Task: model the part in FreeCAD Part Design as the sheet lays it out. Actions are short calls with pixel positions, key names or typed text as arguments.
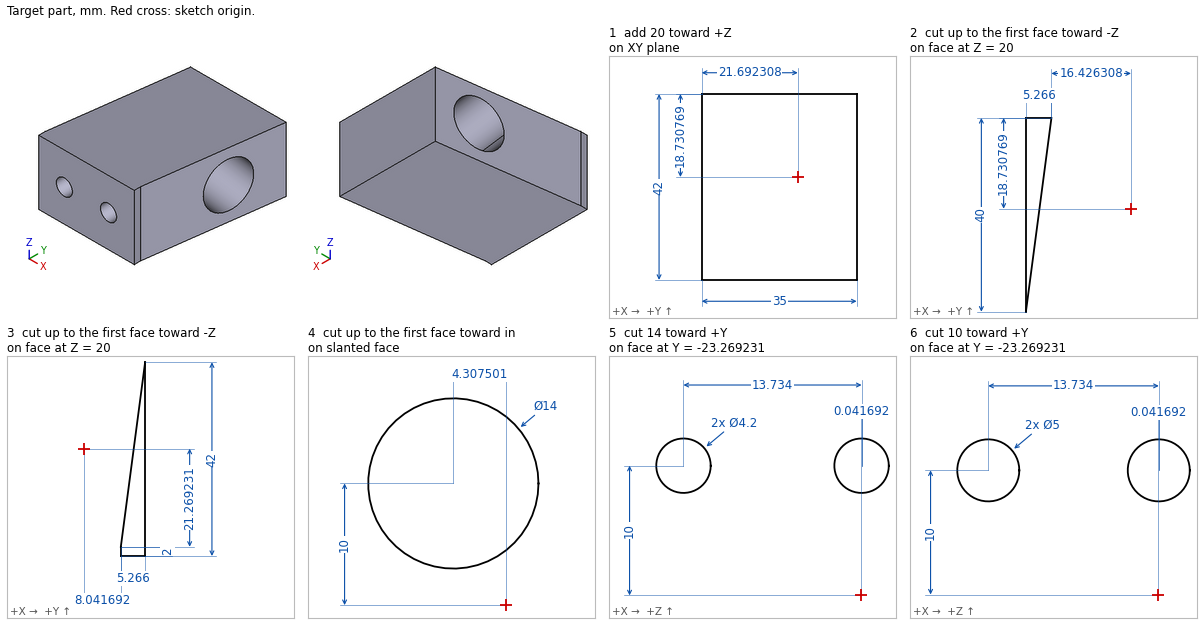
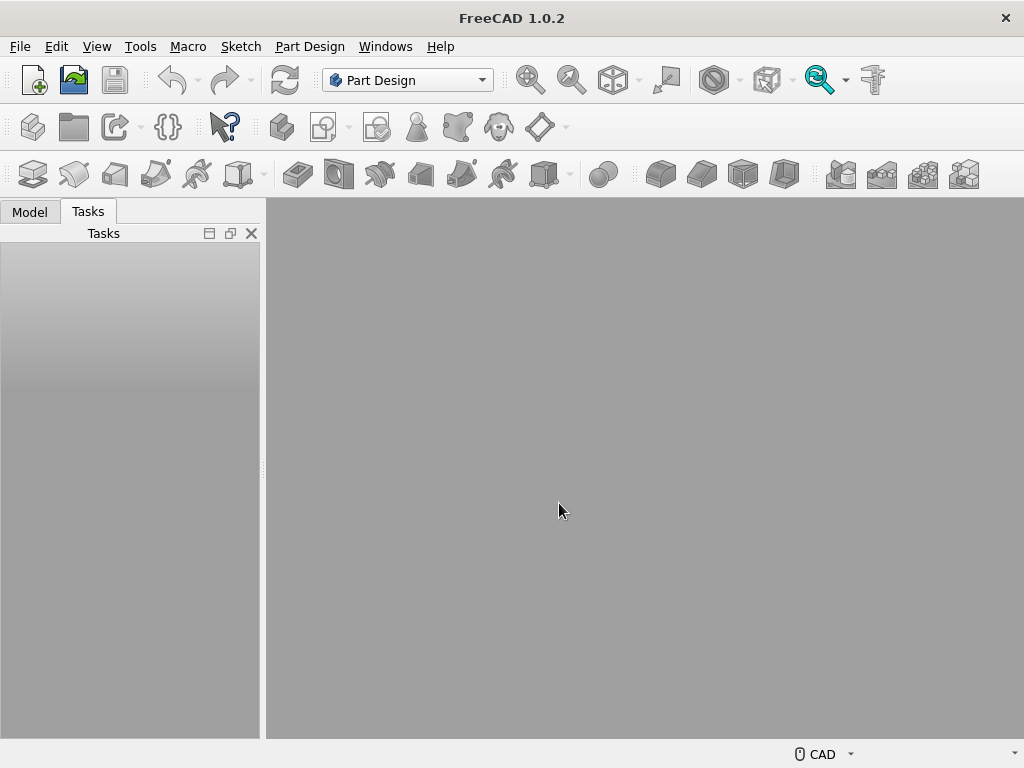
click(33, 80)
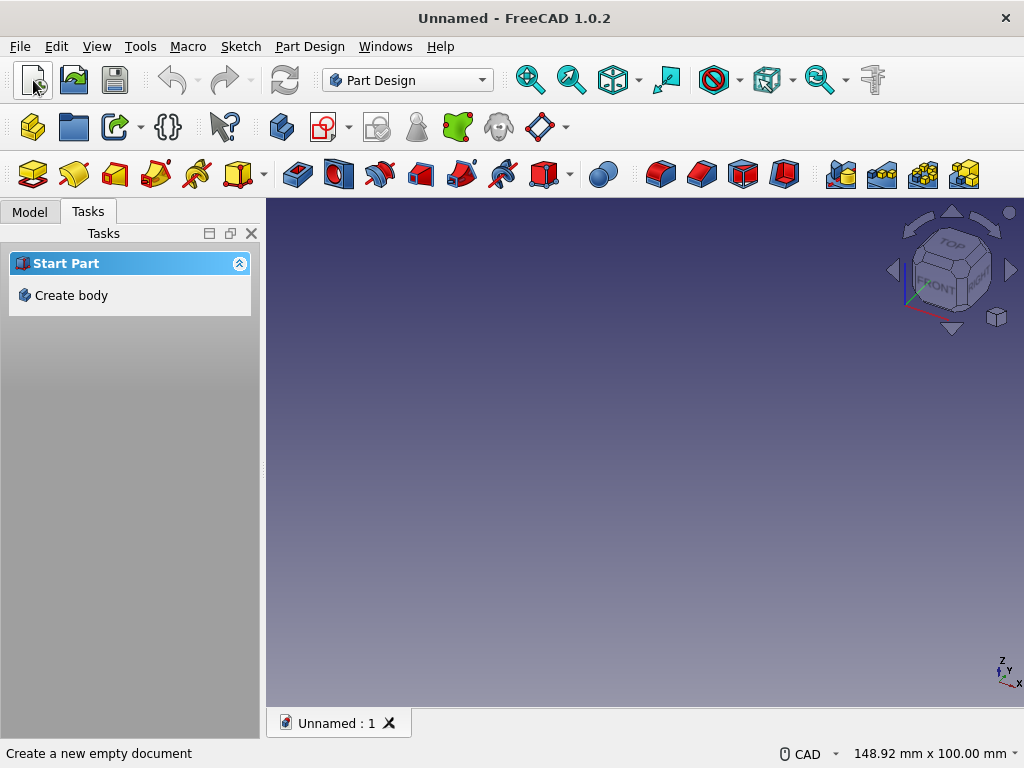
click(322, 128)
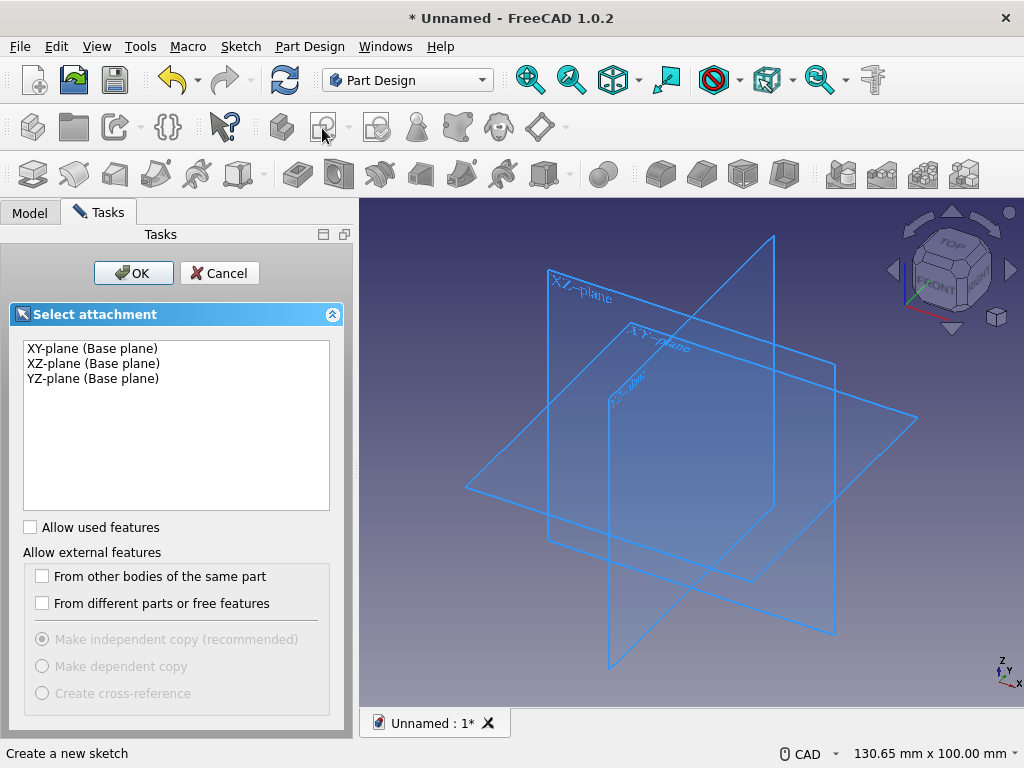
click(84, 348)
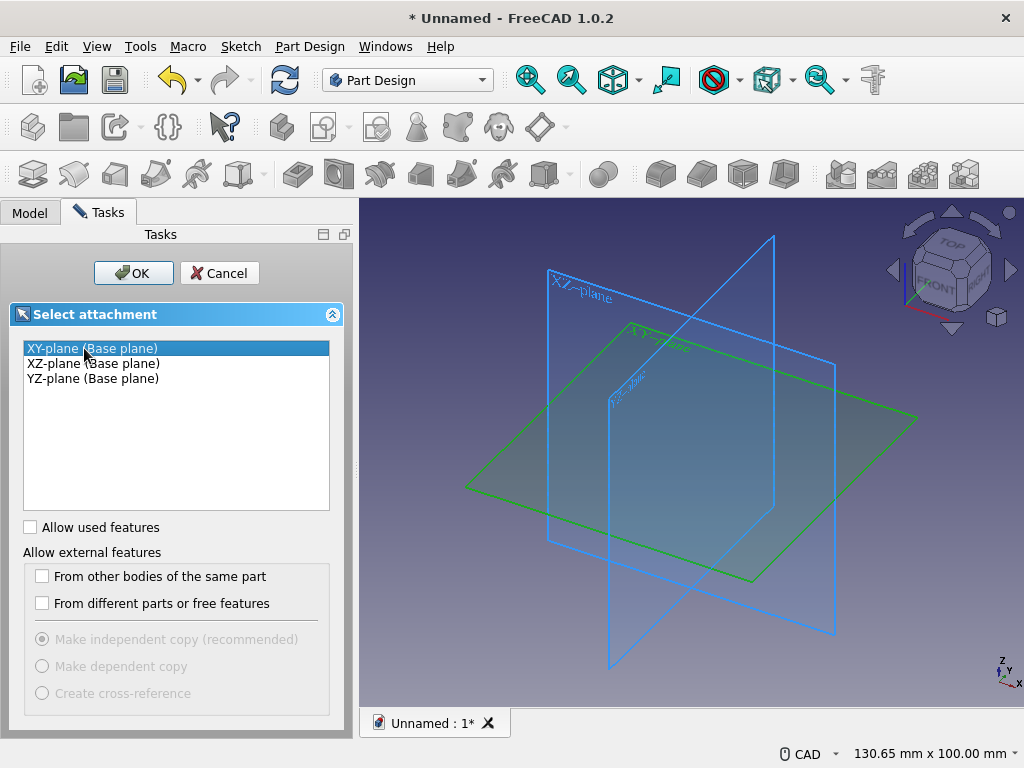
click(134, 273)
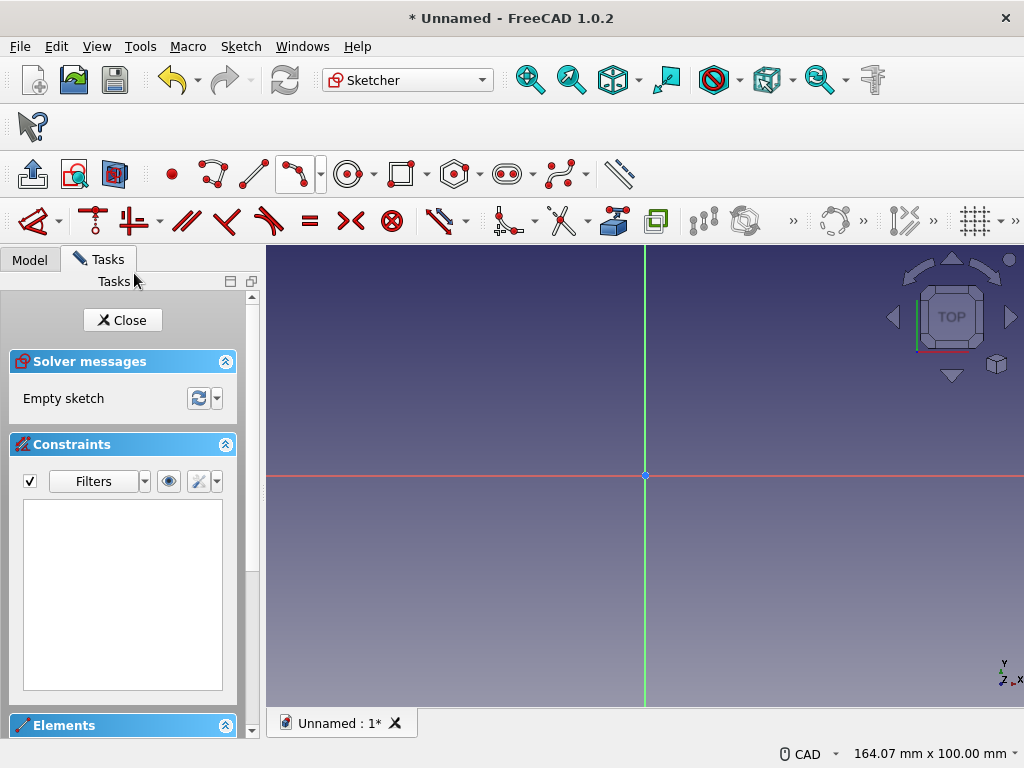
scroll(726, 508, up, 2)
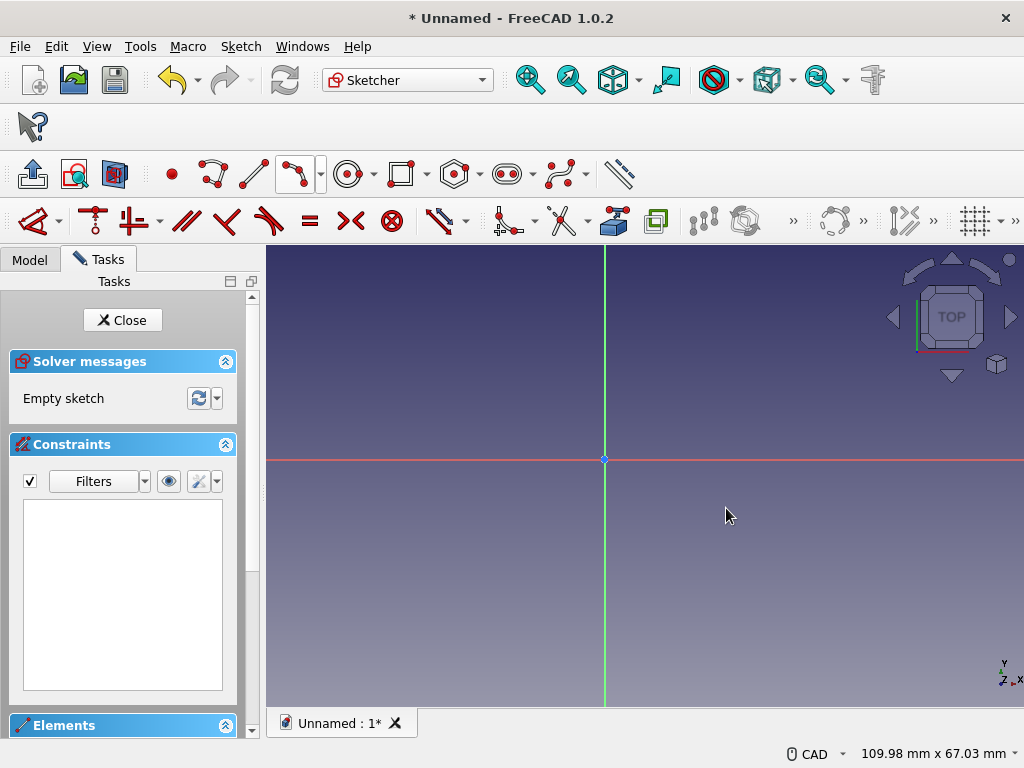
click(400, 174)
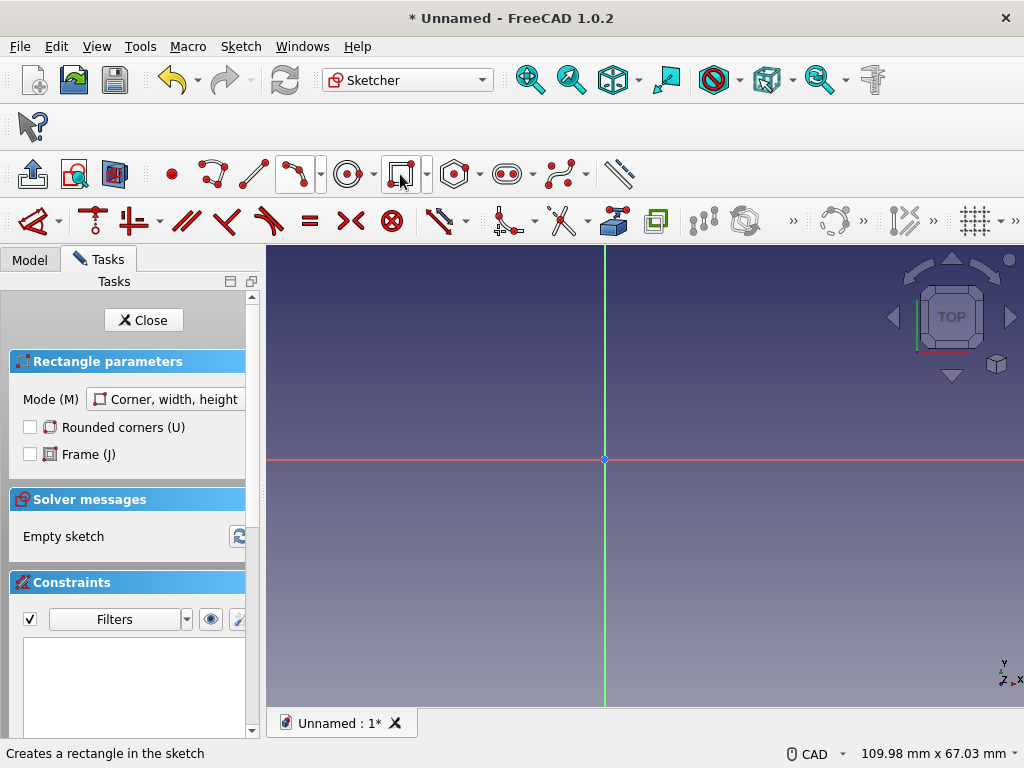
click(455, 331)
click(697, 620)
key(Escape)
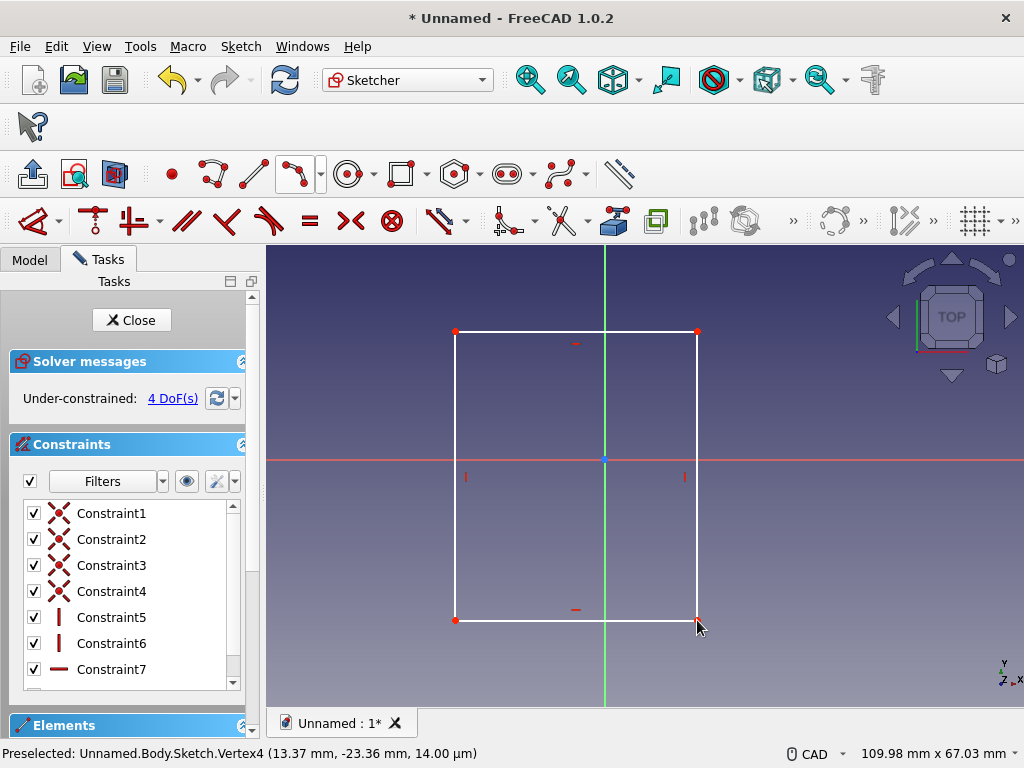
click(32, 222)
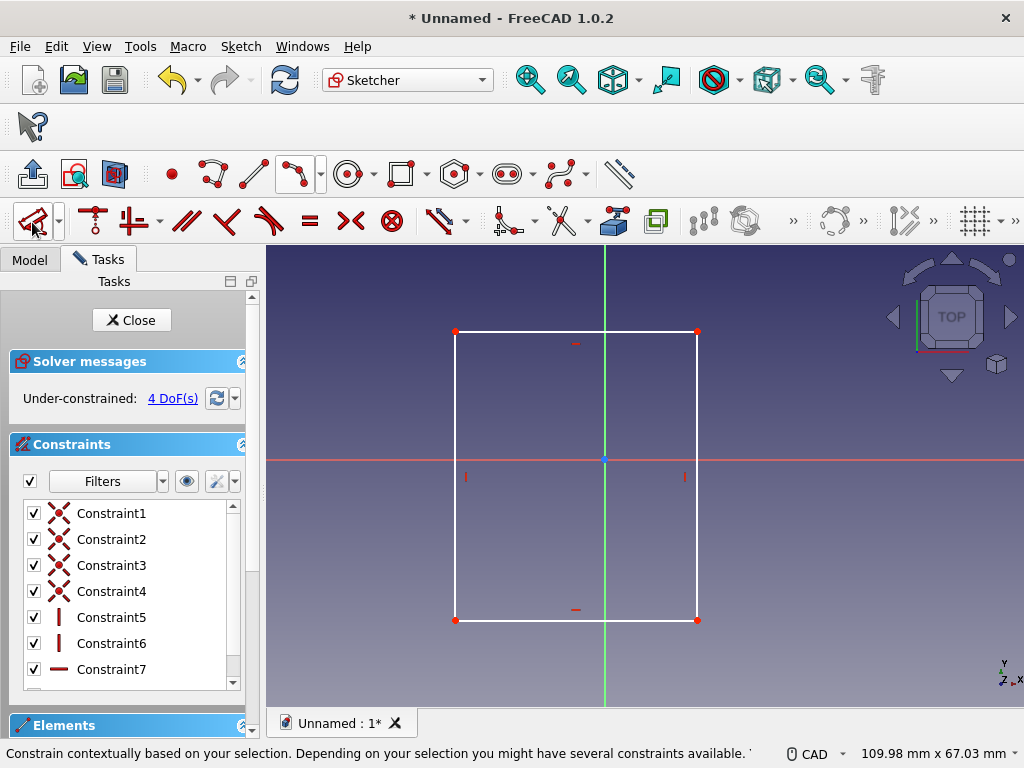
click(455, 419)
click(421, 477)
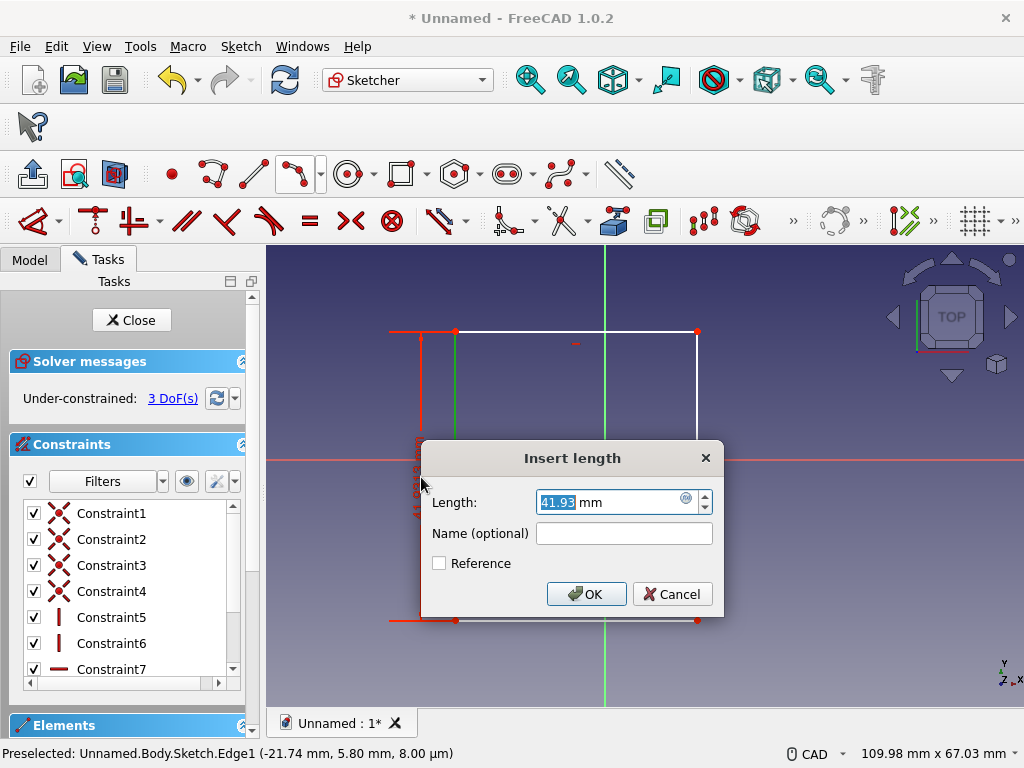
text(42)
key(Return)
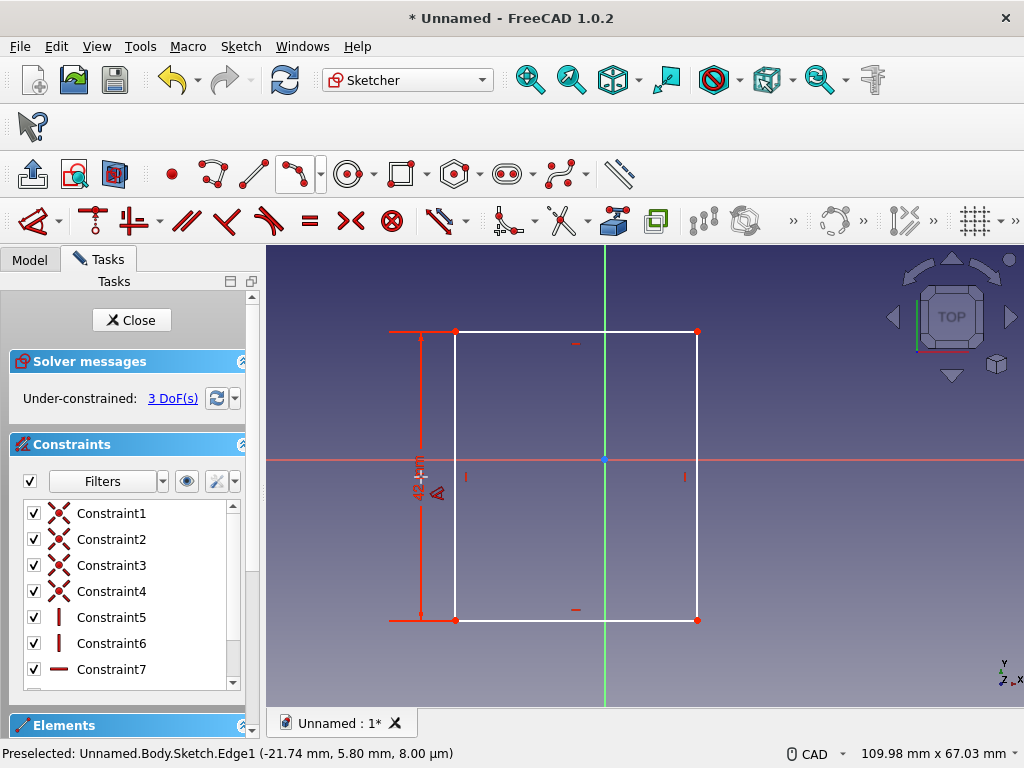
click(528, 621)
click(576, 655)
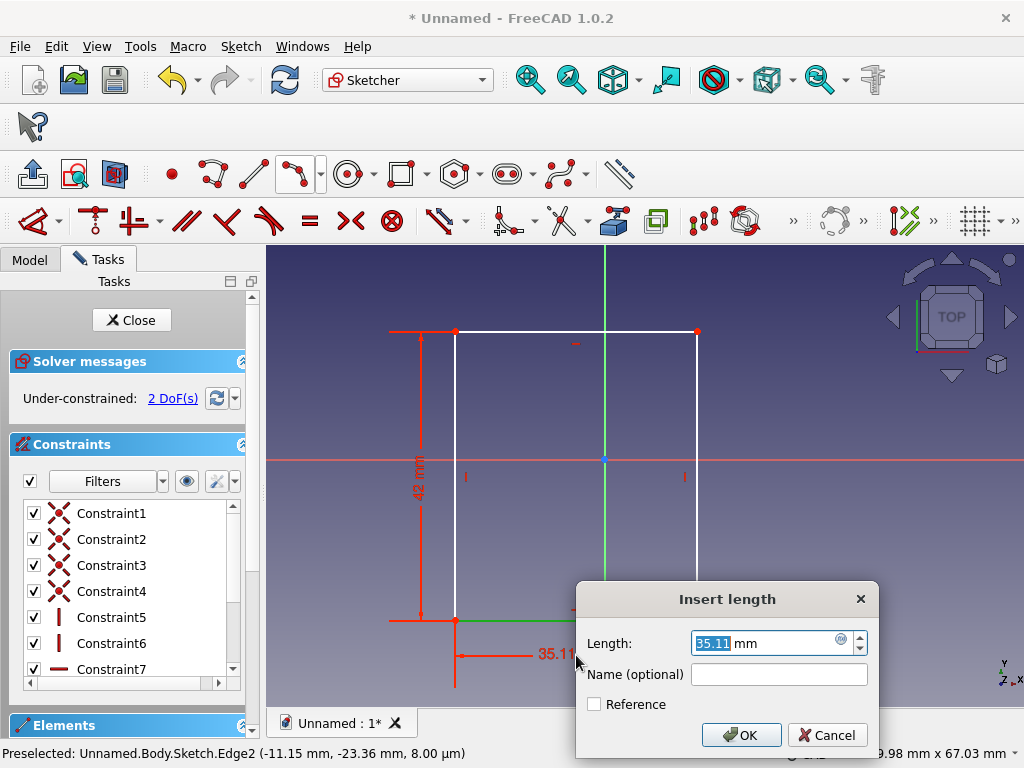
text(35)
key(Return)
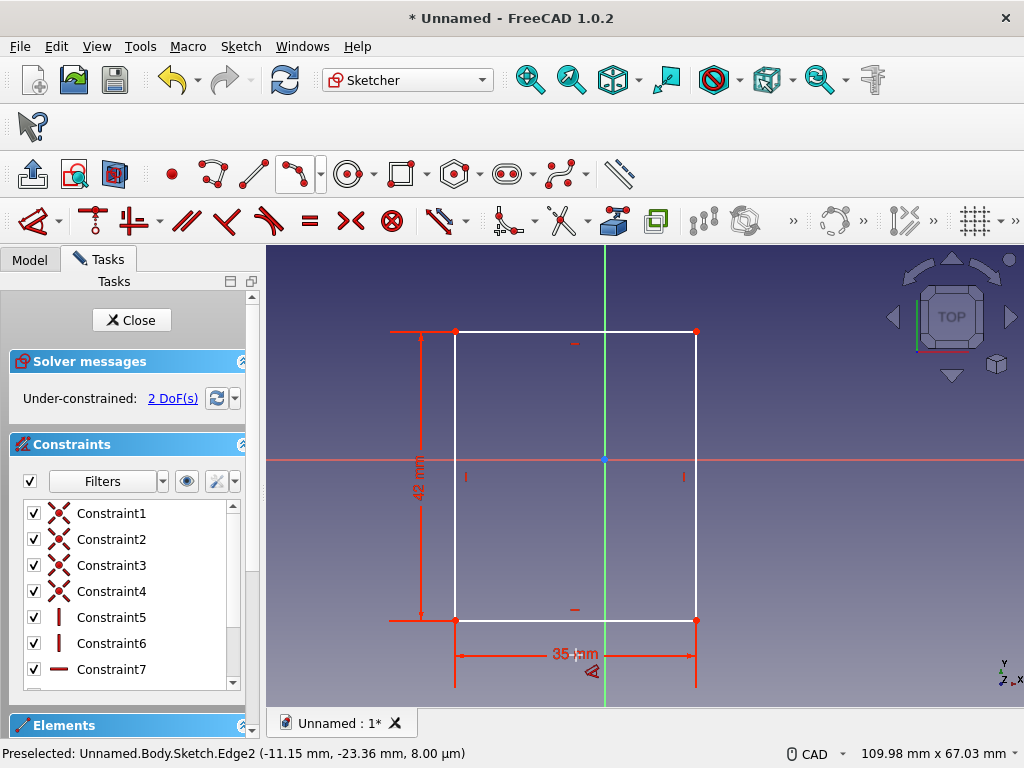
click(455, 332)
click(530, 298)